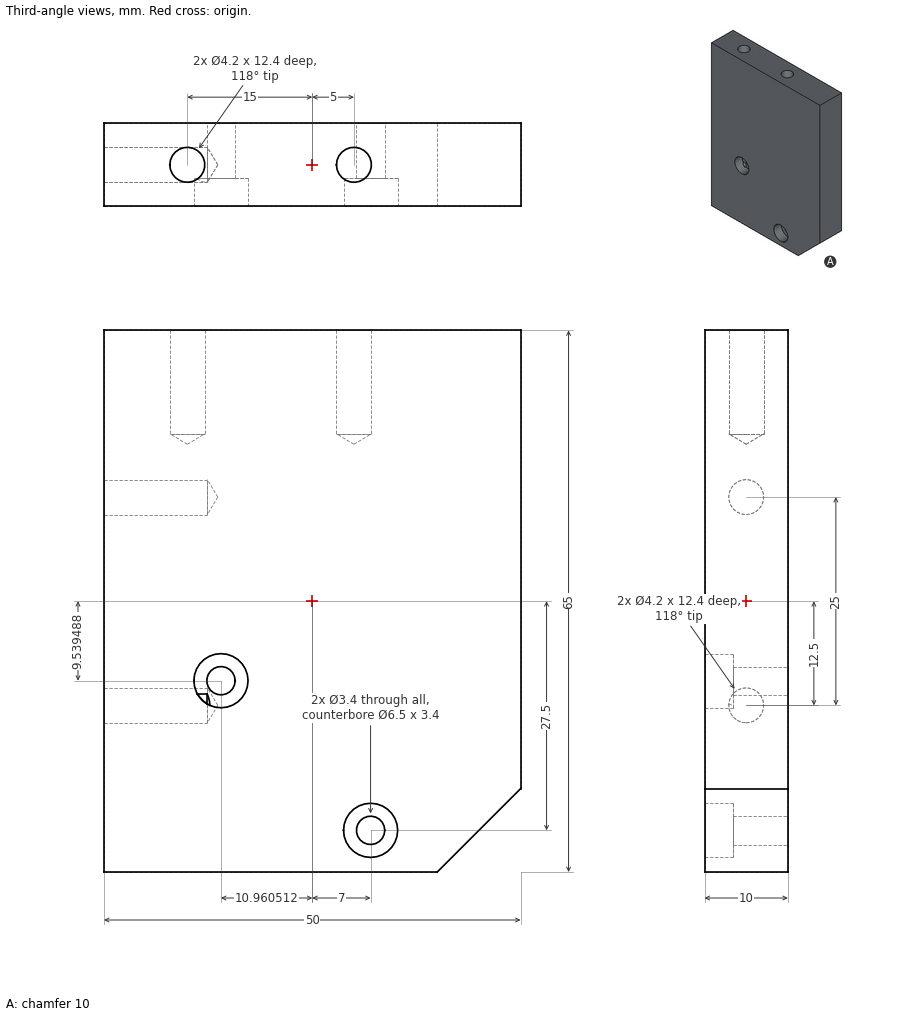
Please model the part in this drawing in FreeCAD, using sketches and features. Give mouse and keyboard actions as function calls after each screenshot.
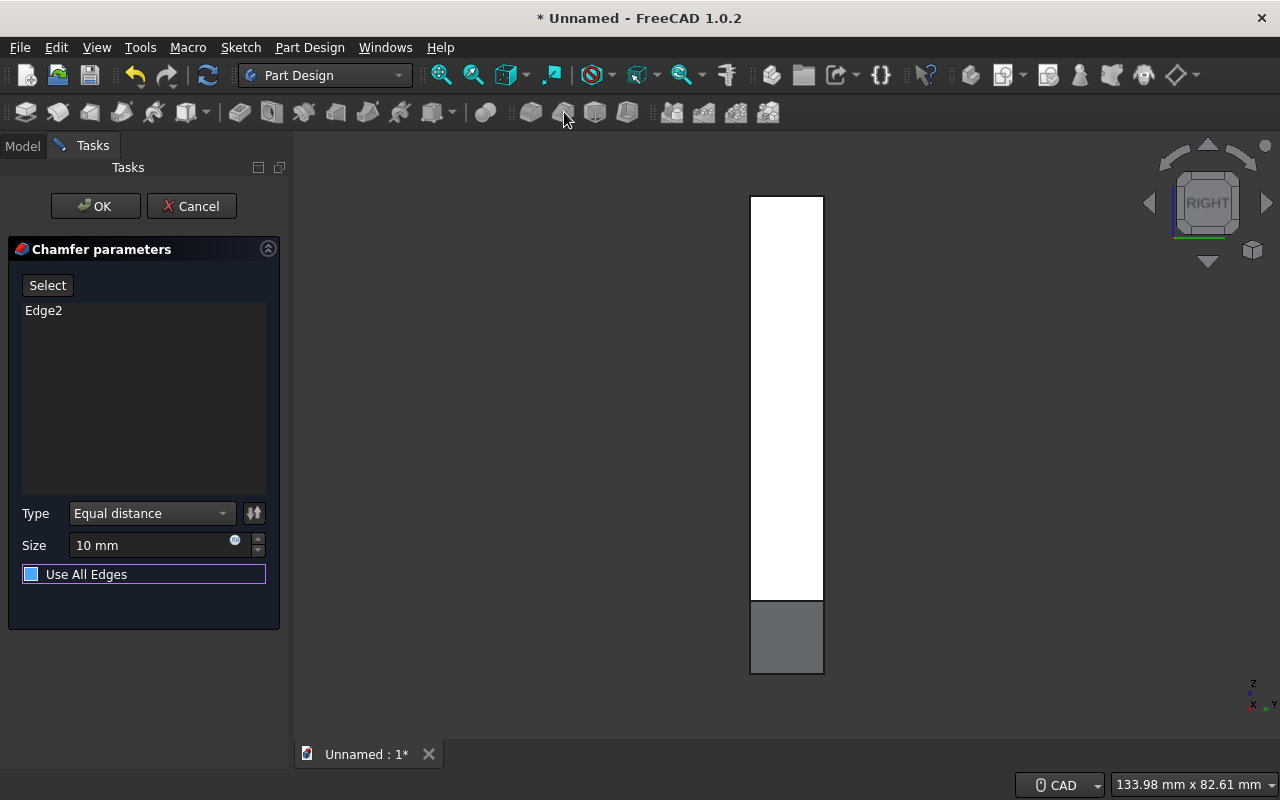
click(96, 206)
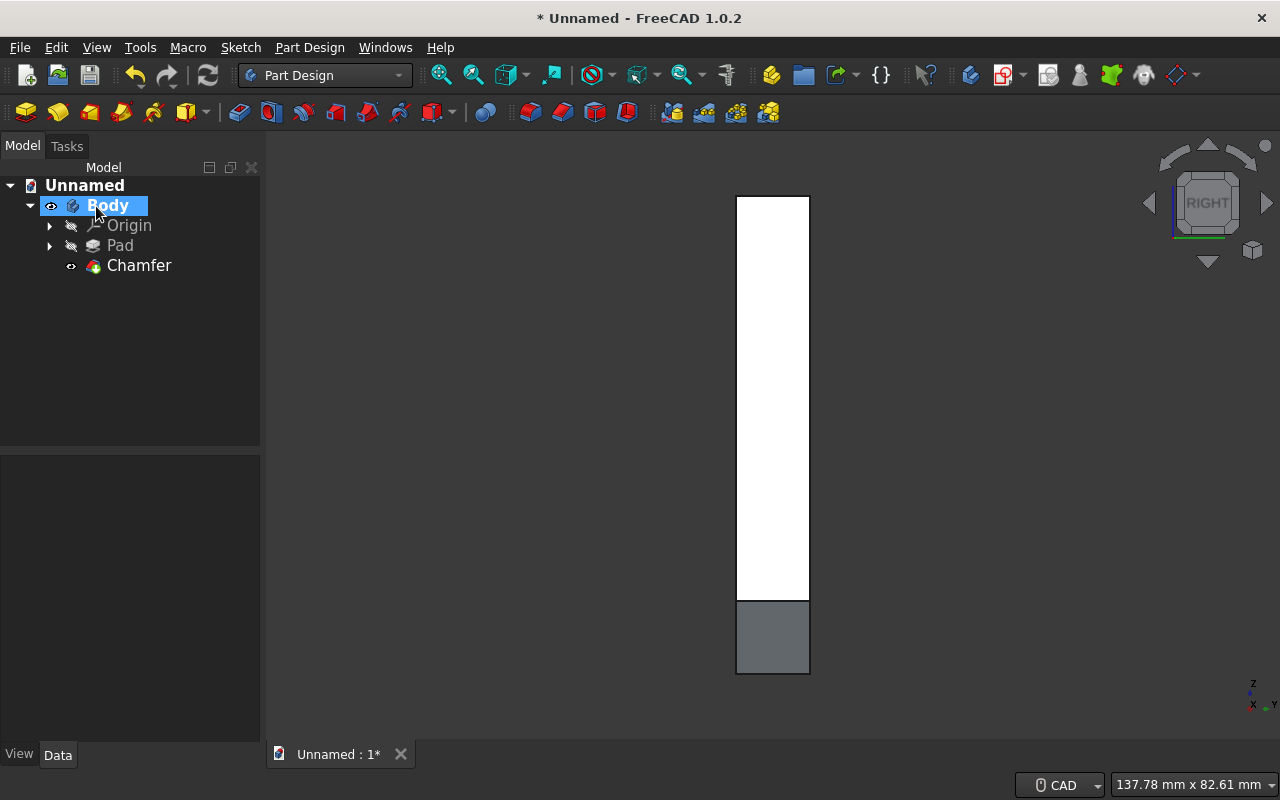
key(6)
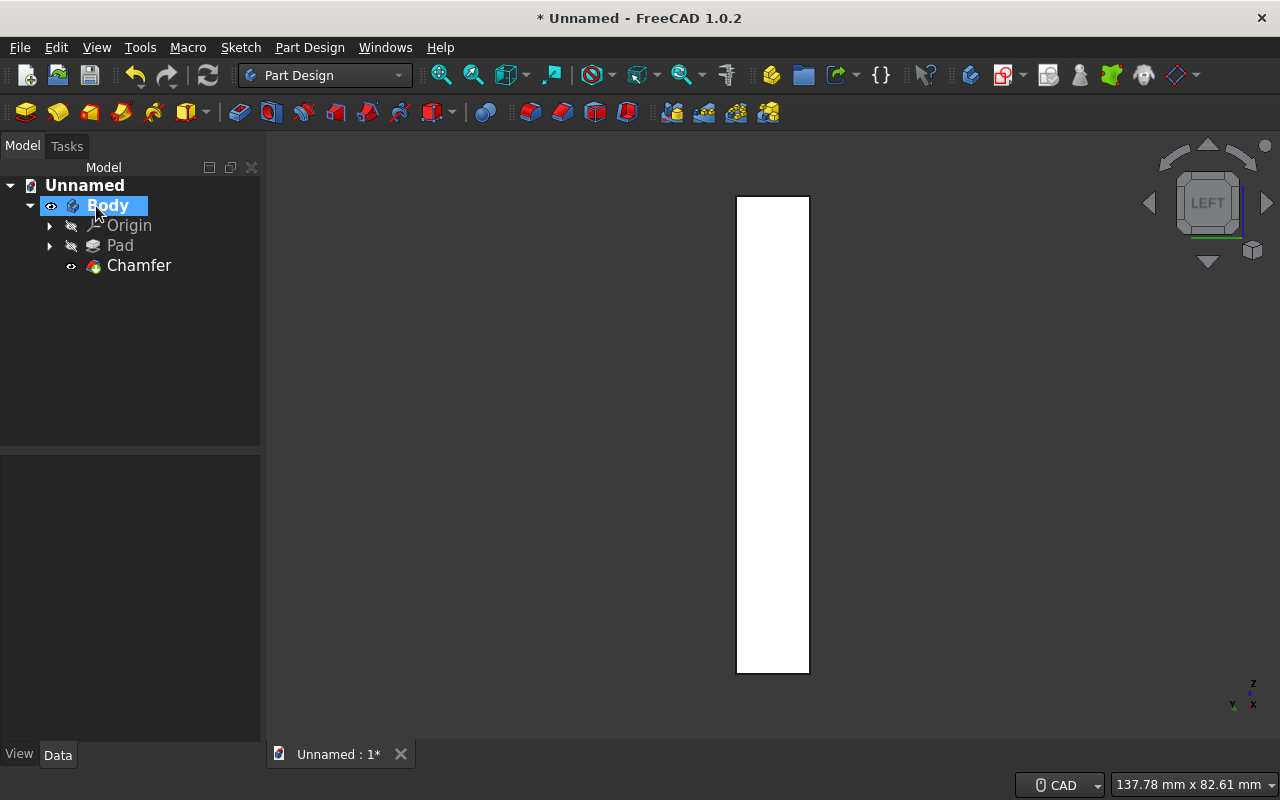
click(773, 366)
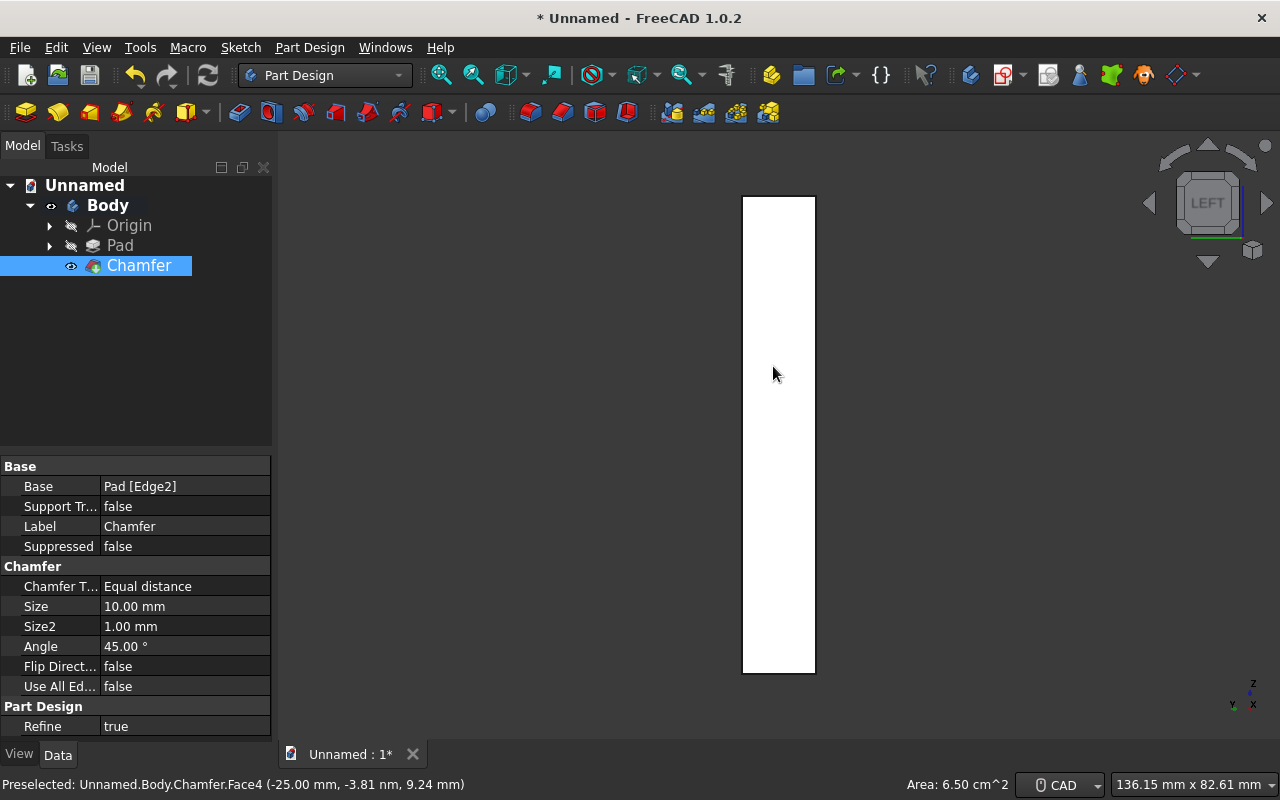
click(1004, 76)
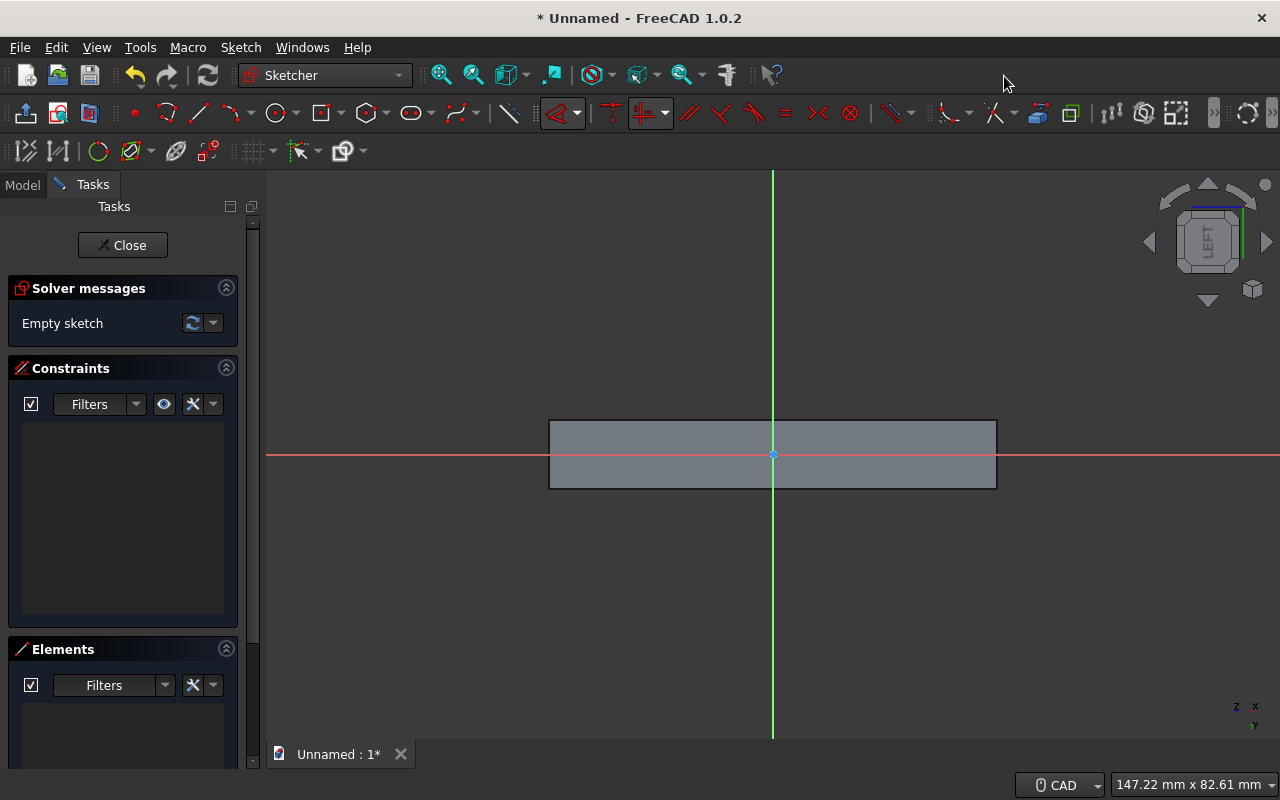
scroll(813, 455, up, 5)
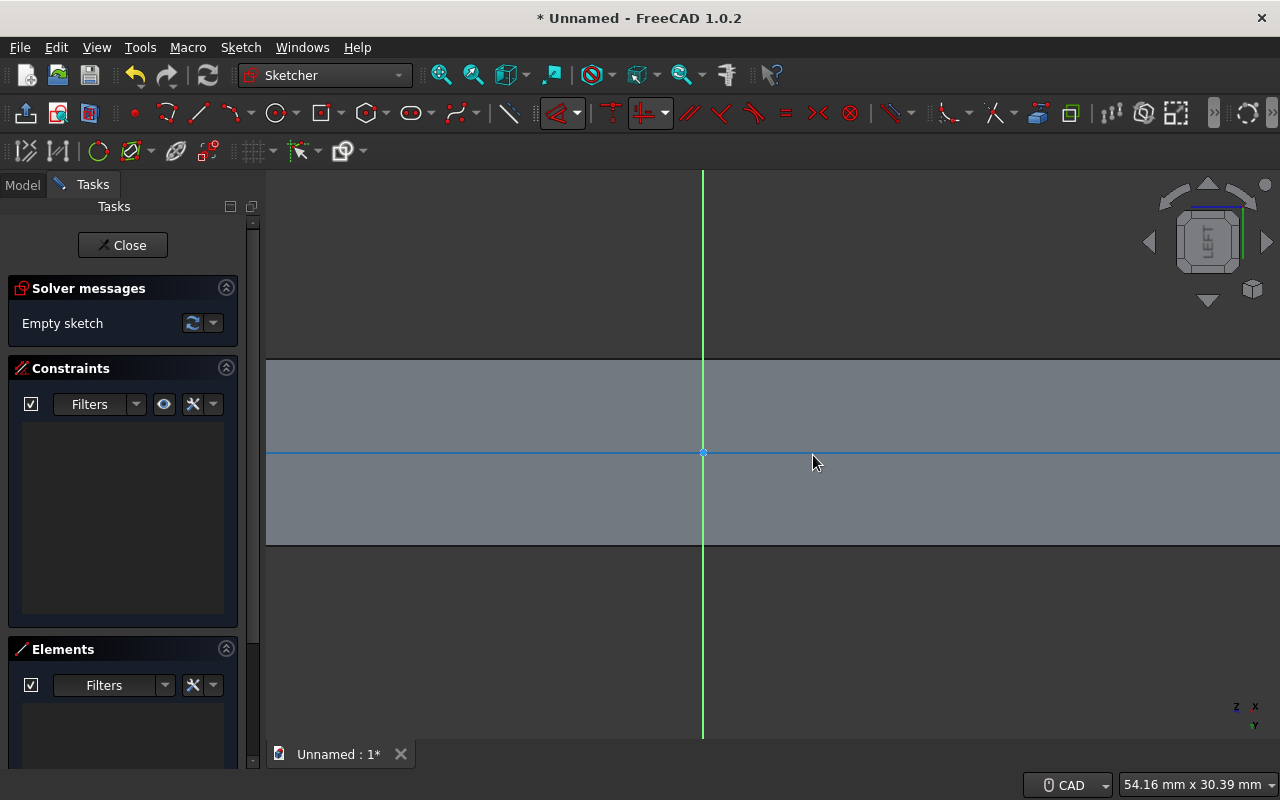
click(276, 114)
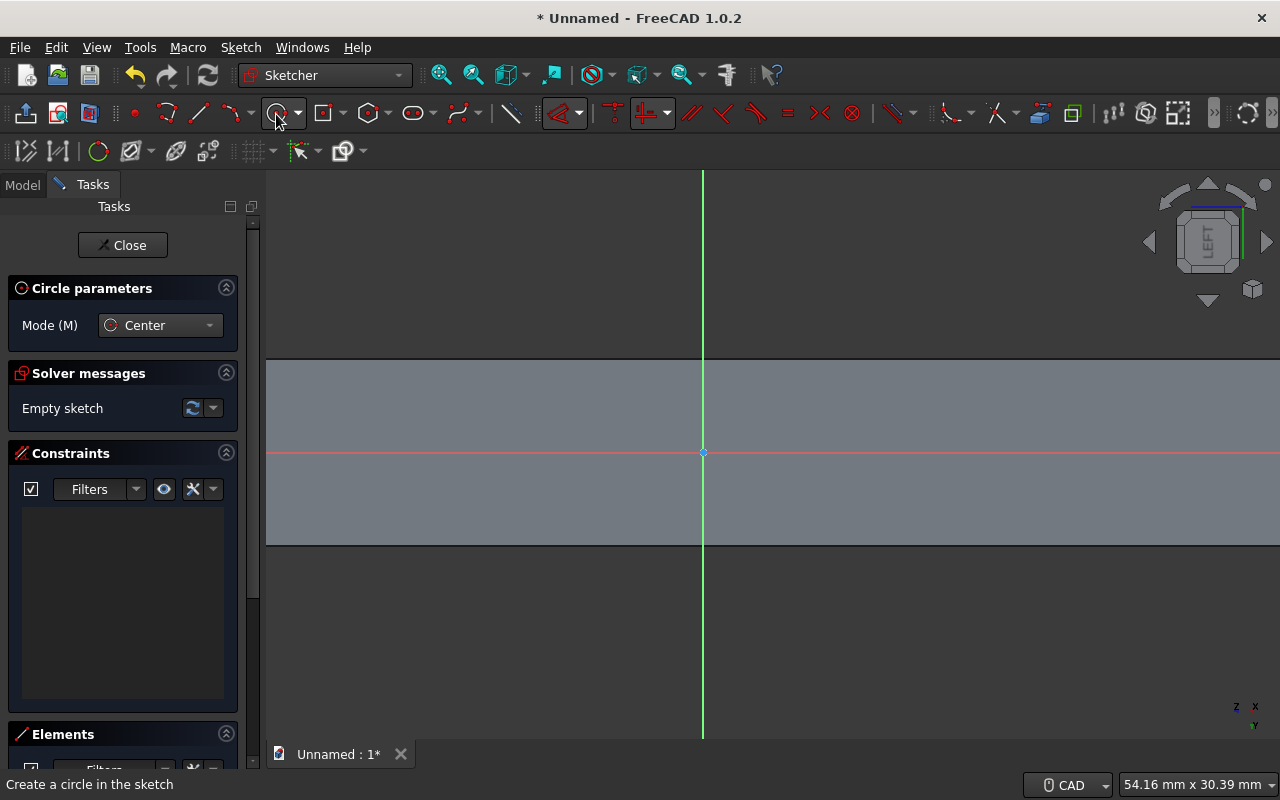
click(937, 453)
move(965, 425)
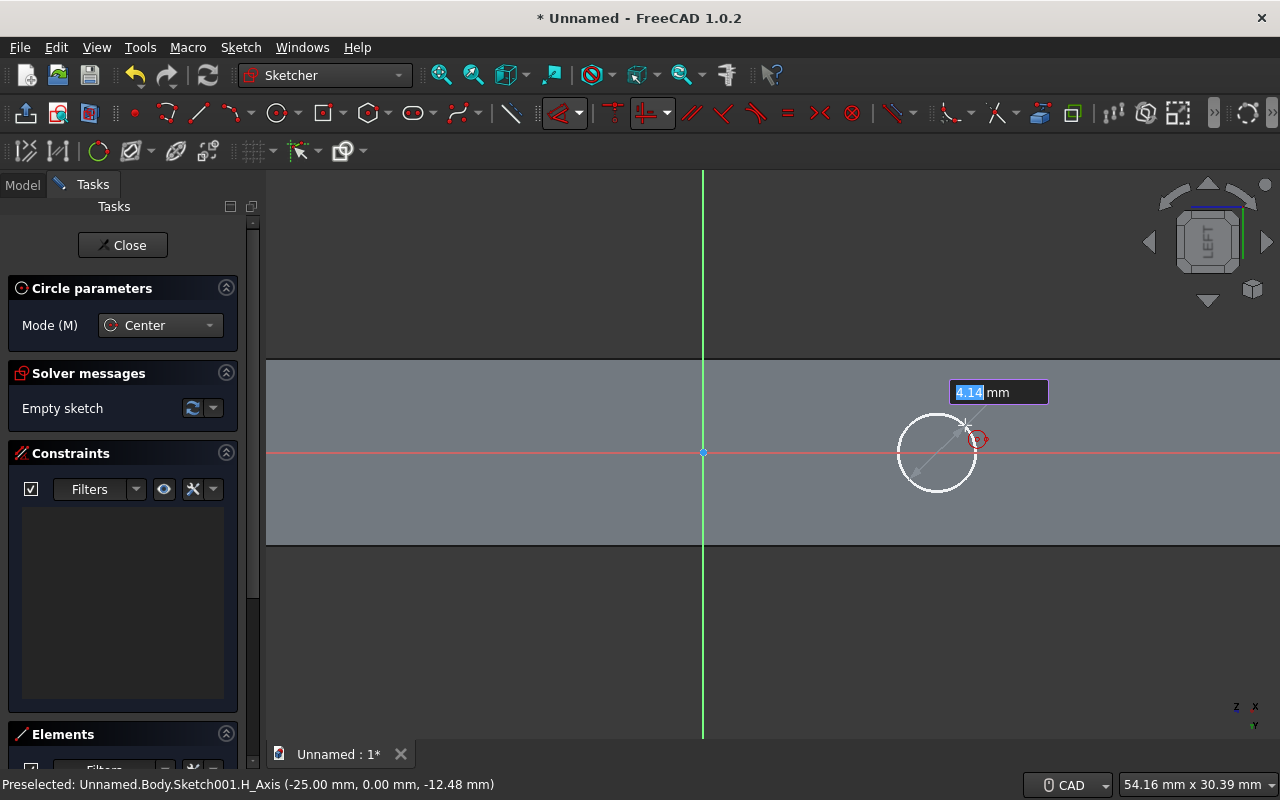
text(4.2)
key(Return)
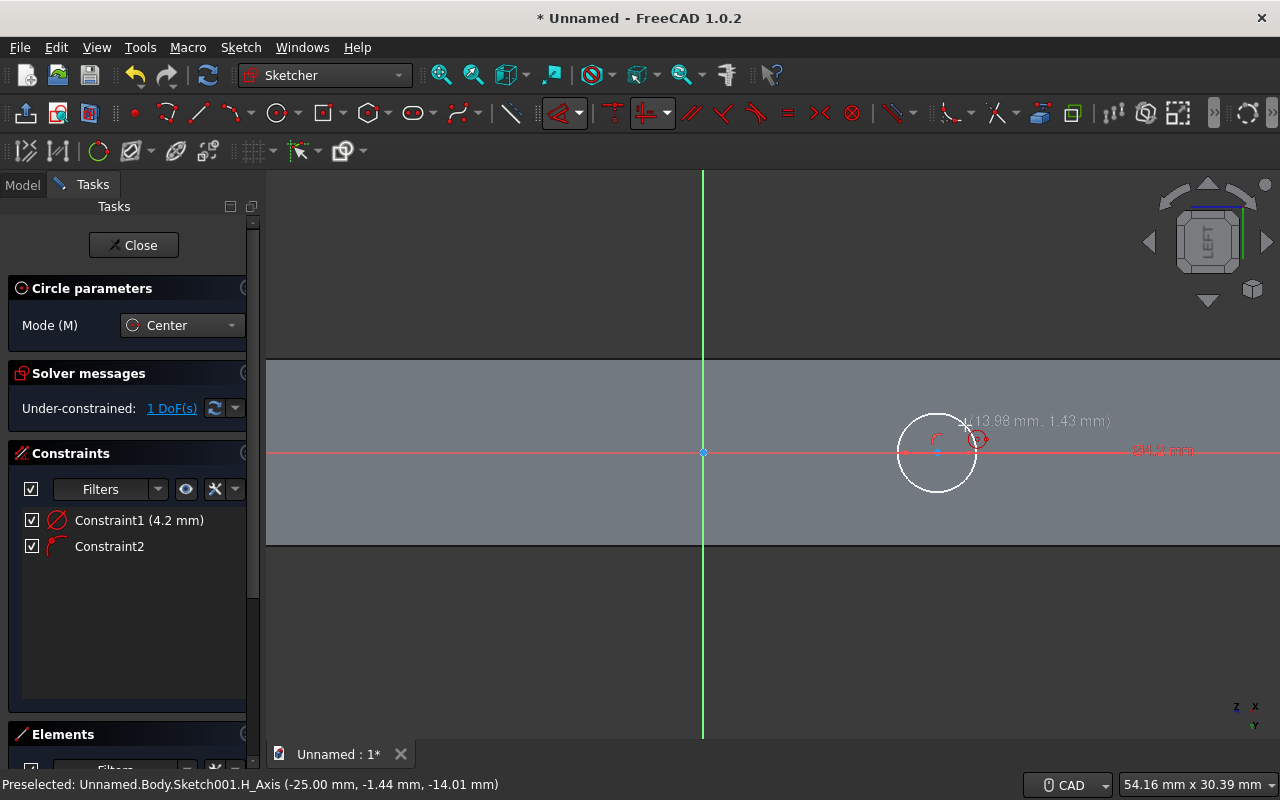
click(469, 453)
move(497, 425)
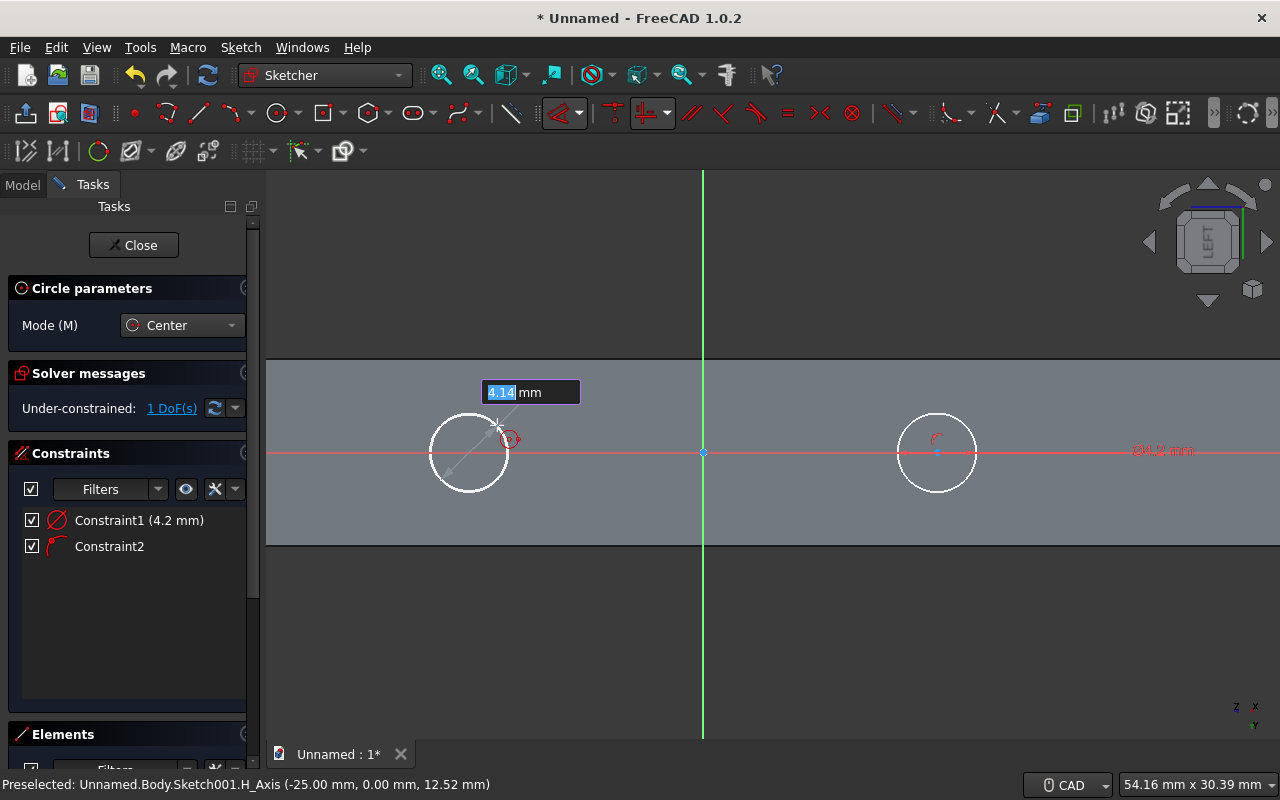
text(4.2)
key(Return)
key(Escape)